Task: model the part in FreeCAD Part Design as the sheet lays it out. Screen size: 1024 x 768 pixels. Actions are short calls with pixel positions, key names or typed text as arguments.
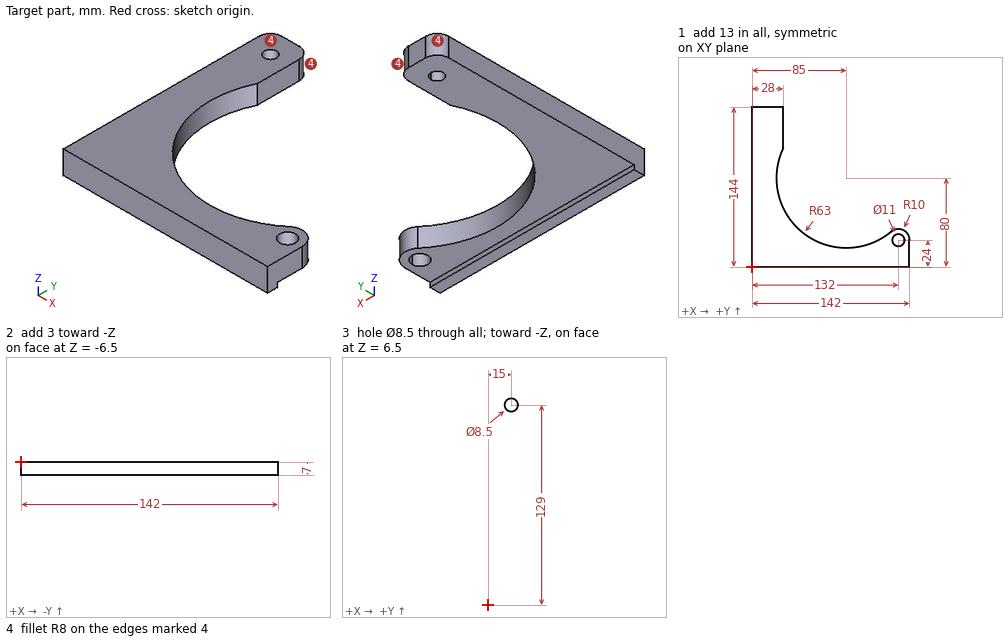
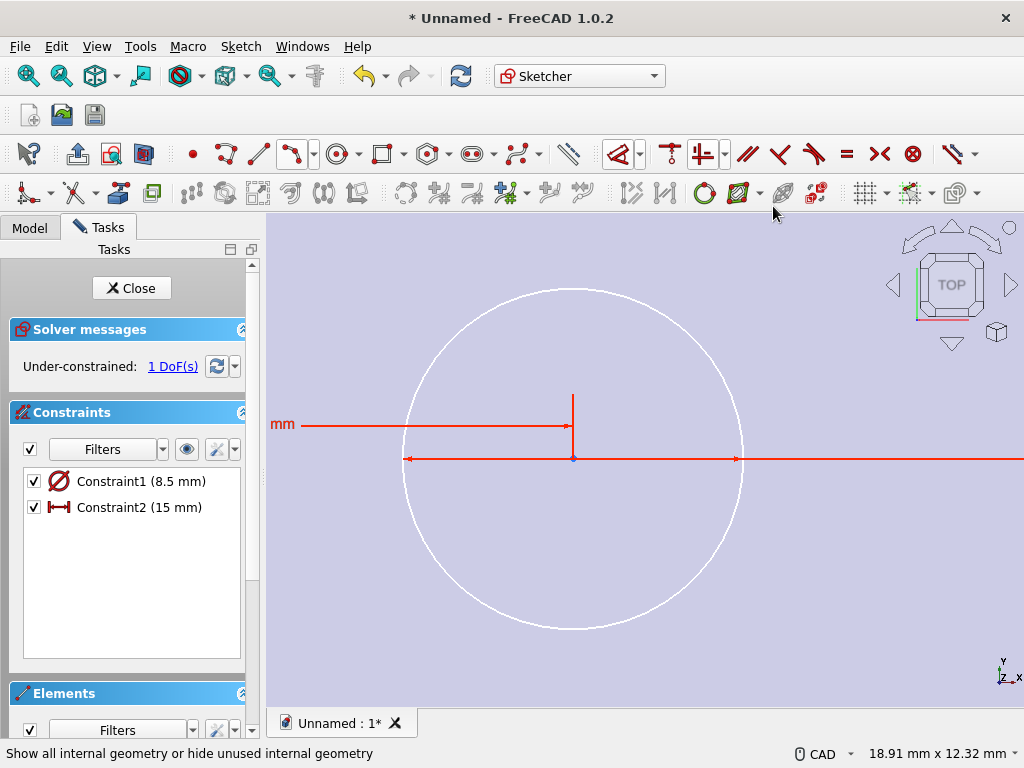
click(573, 459)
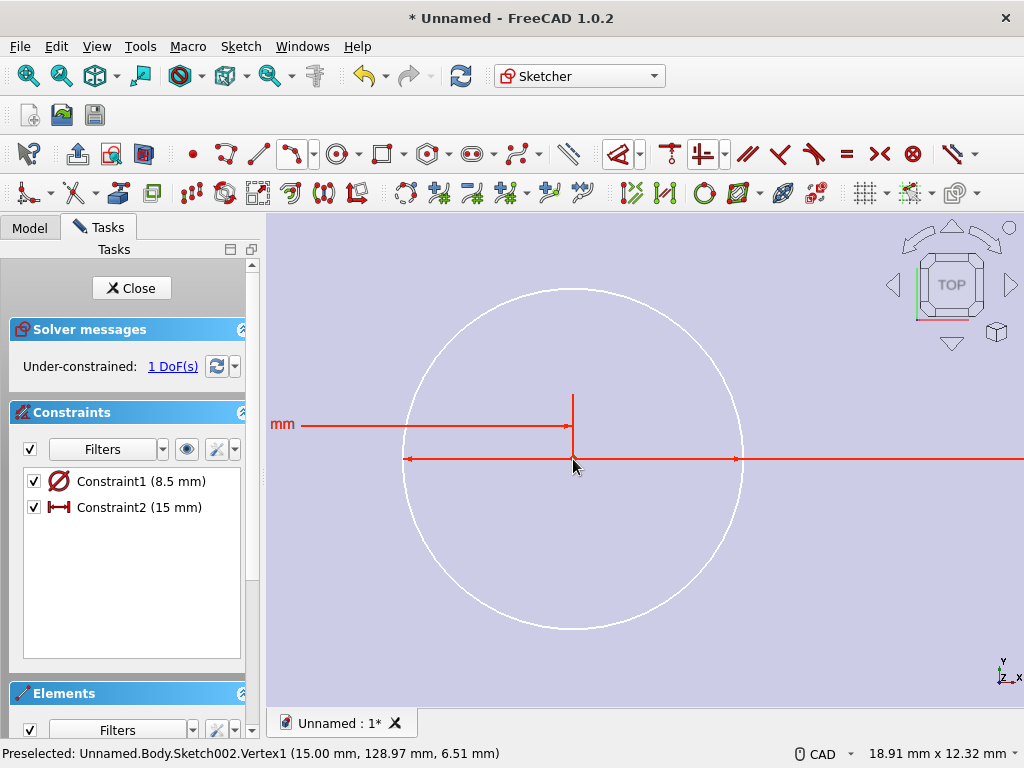
click(640, 154)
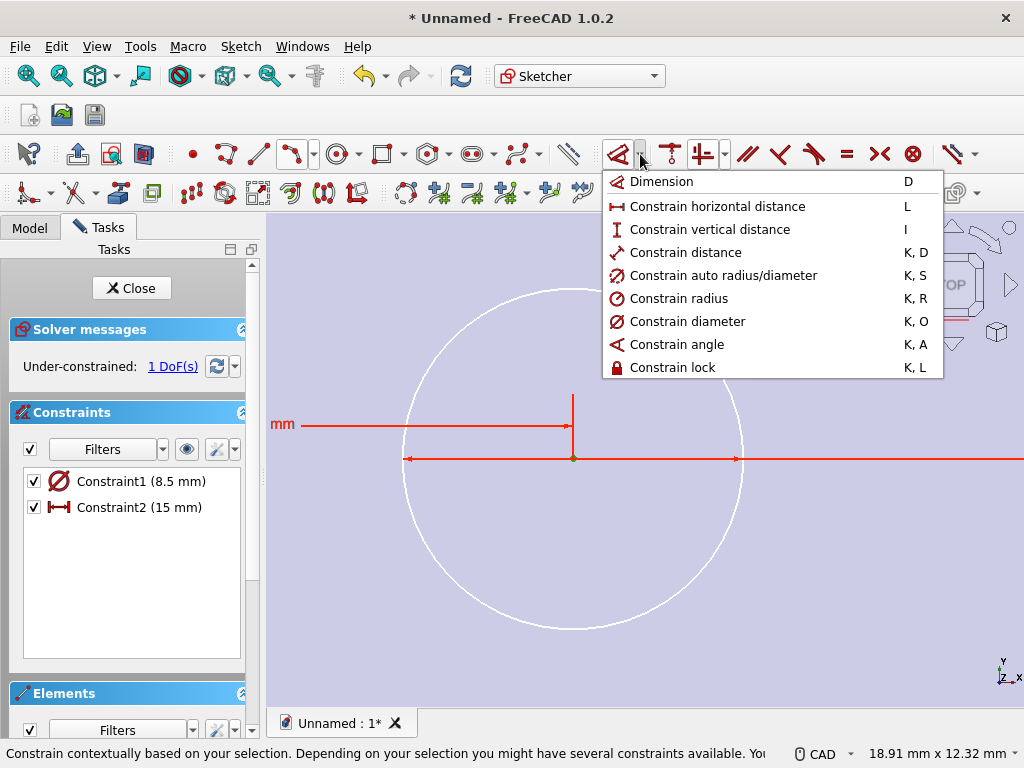
click(773, 230)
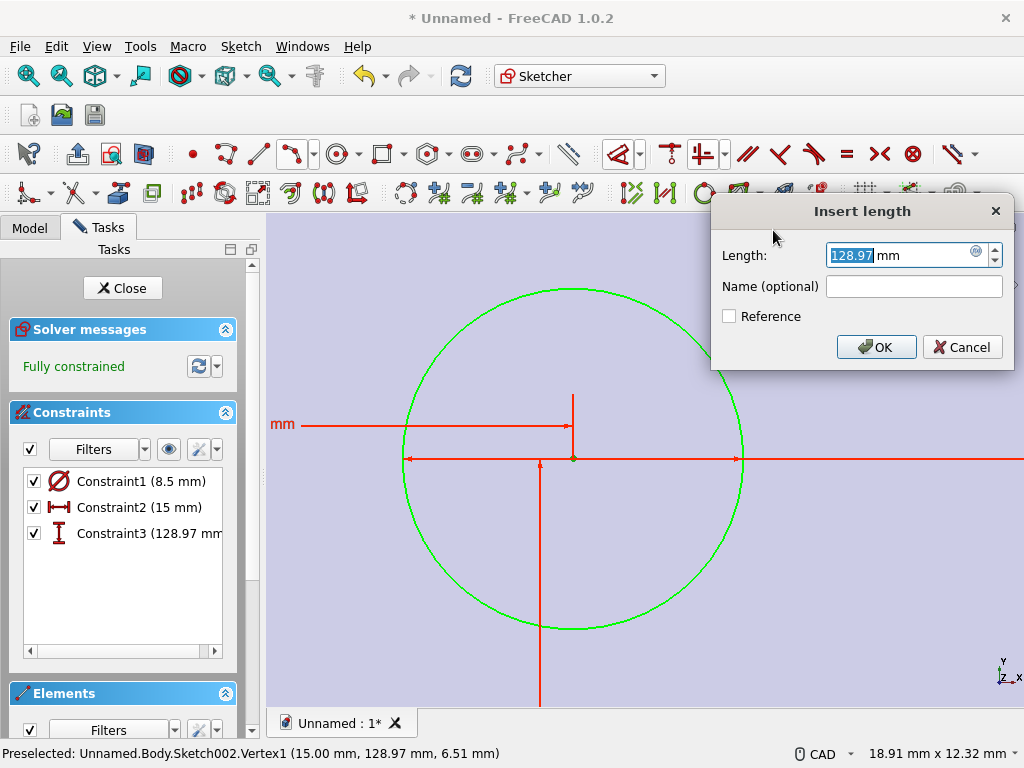
text(129)
key(Return)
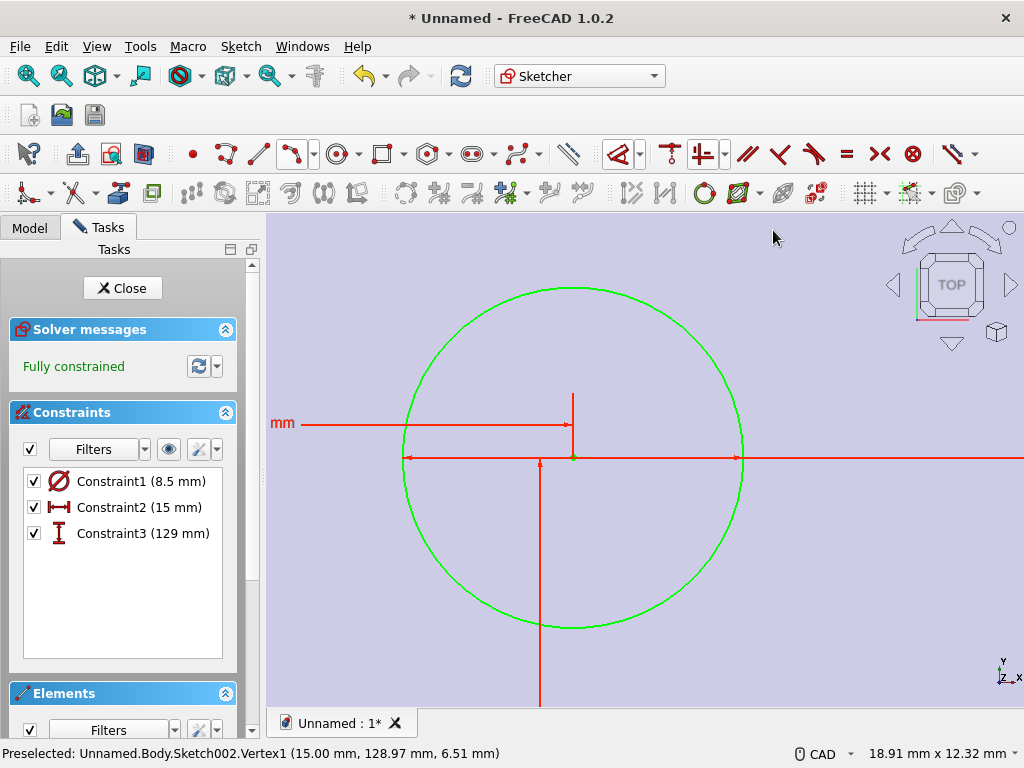
click(123, 288)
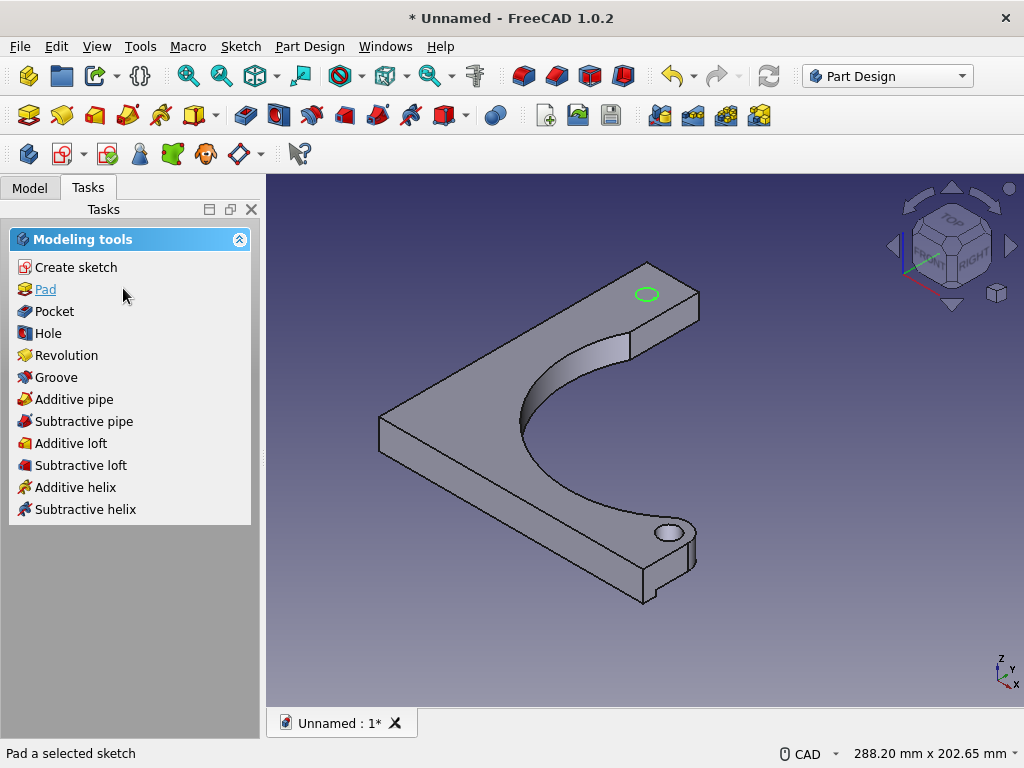
click(279, 116)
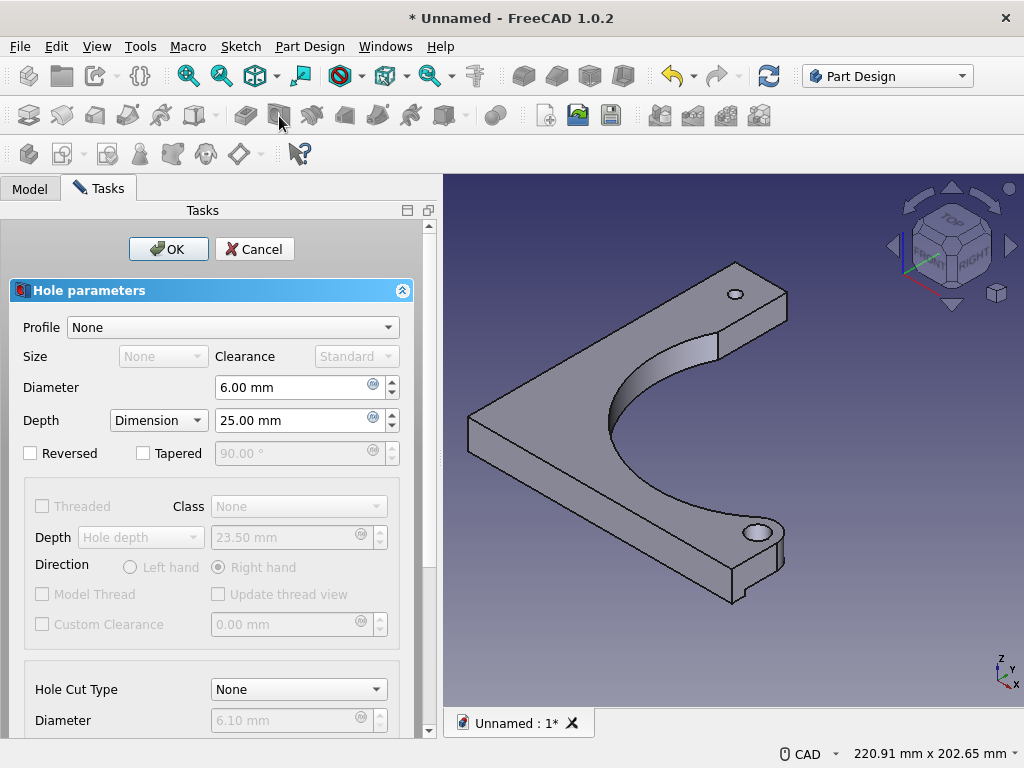
triple_click(300, 388)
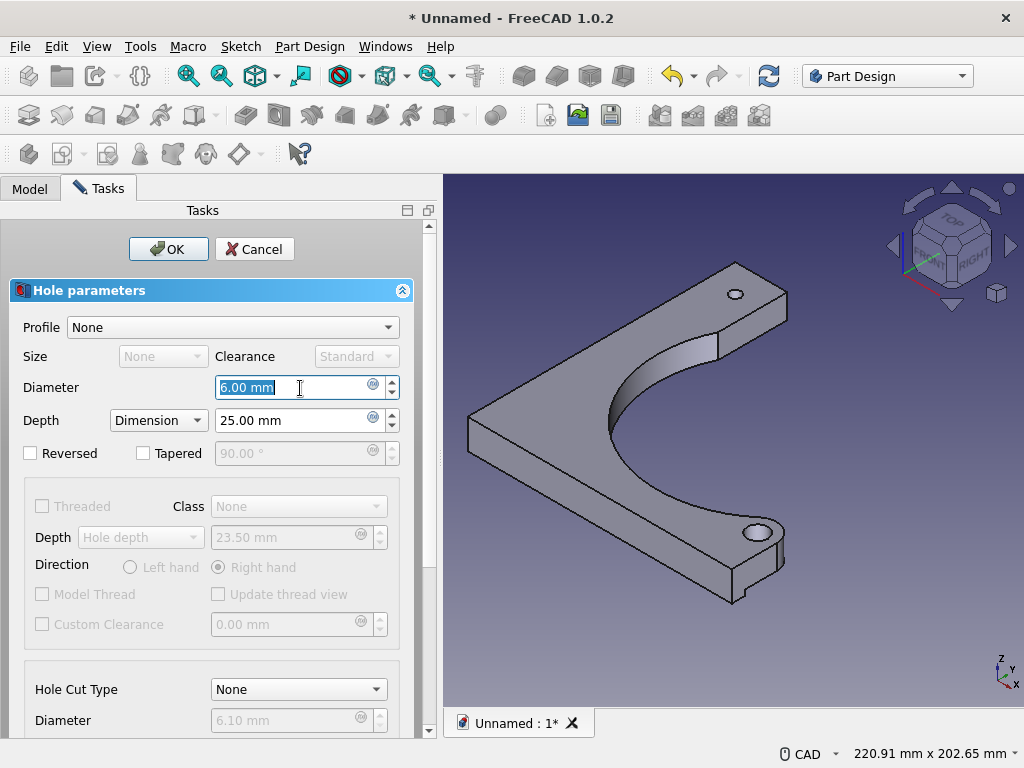
text(8.5)
key(Tab)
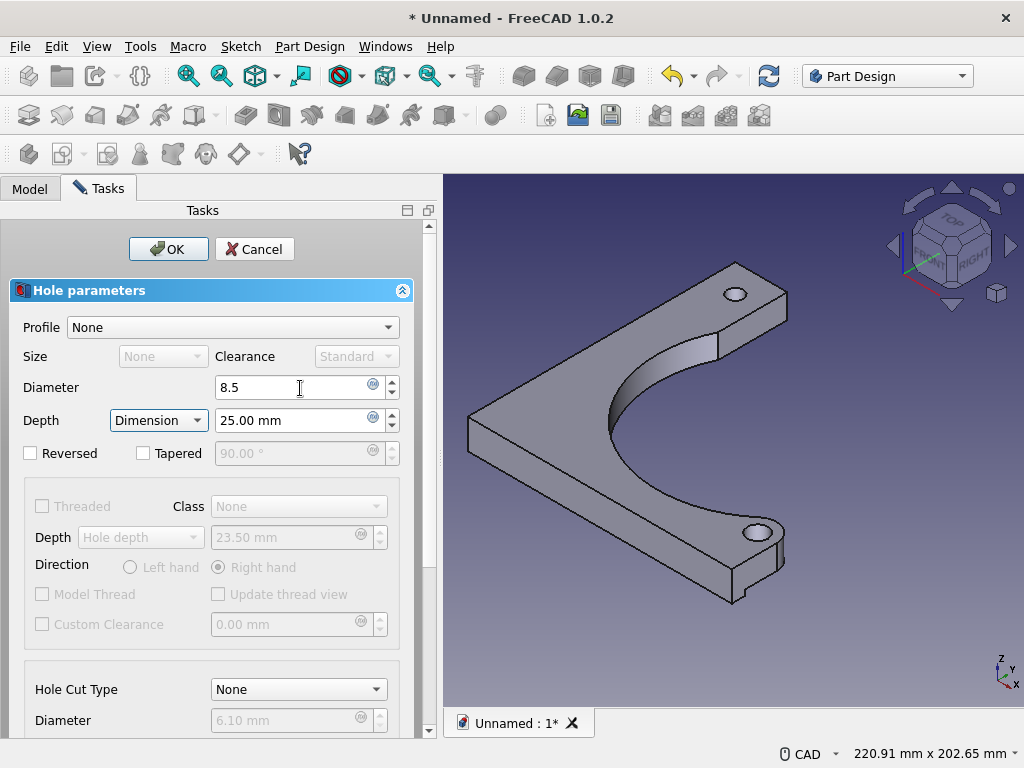
click(160, 420)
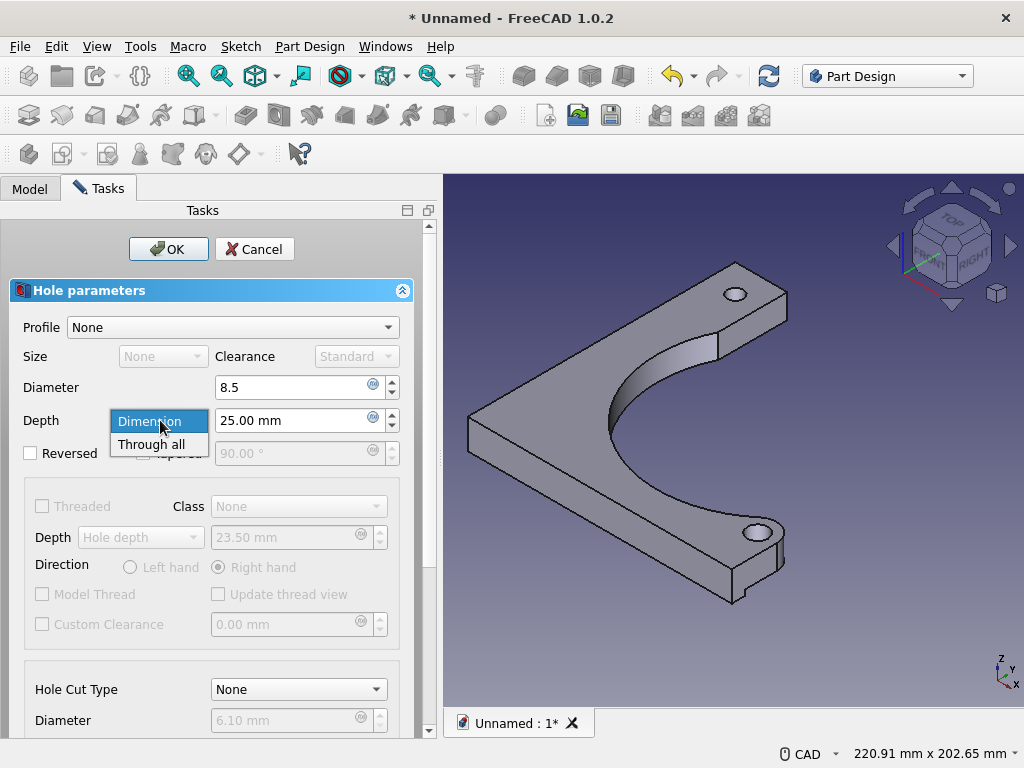
click(158, 444)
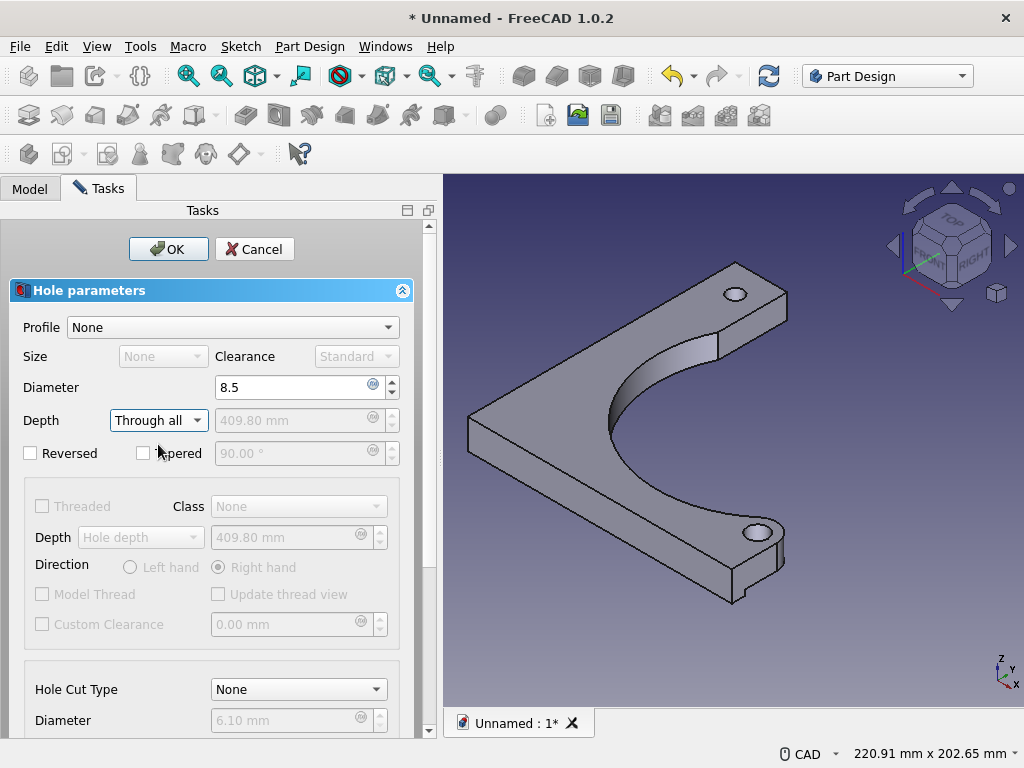
click(169, 249)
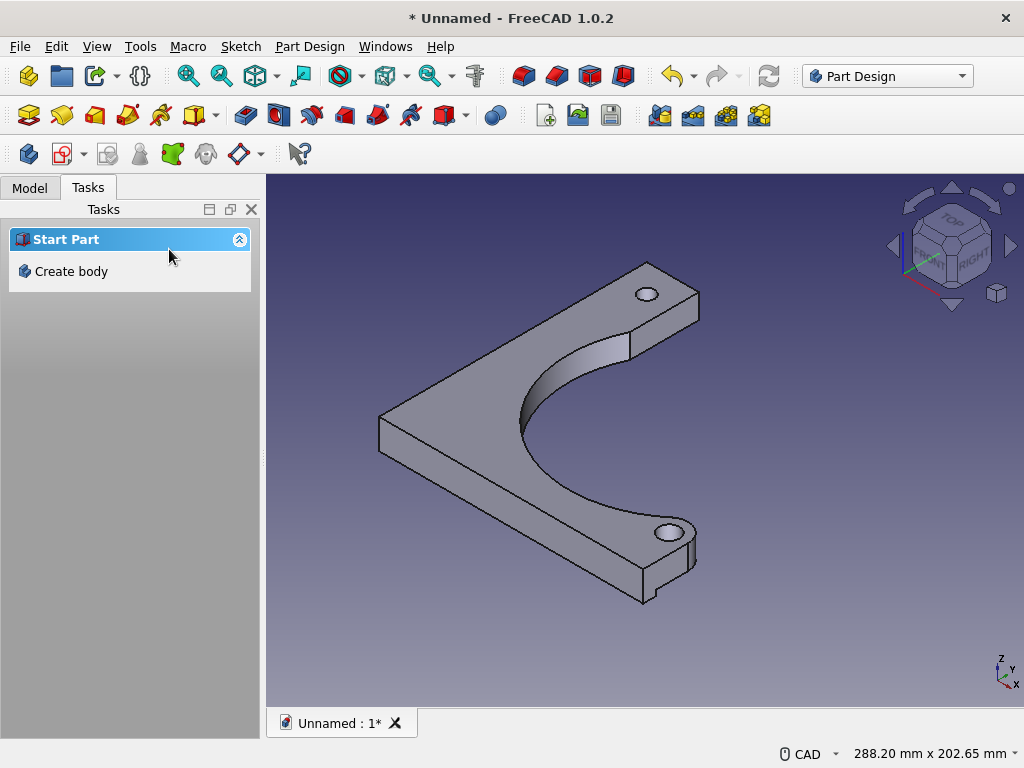
key(2)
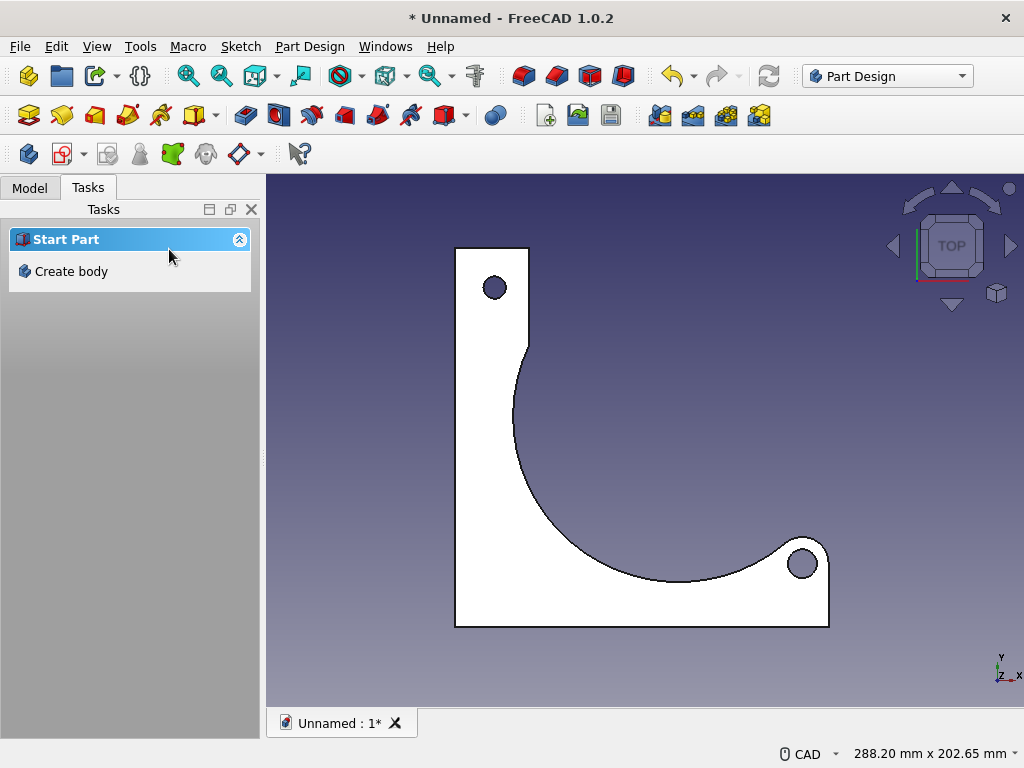
key(0)